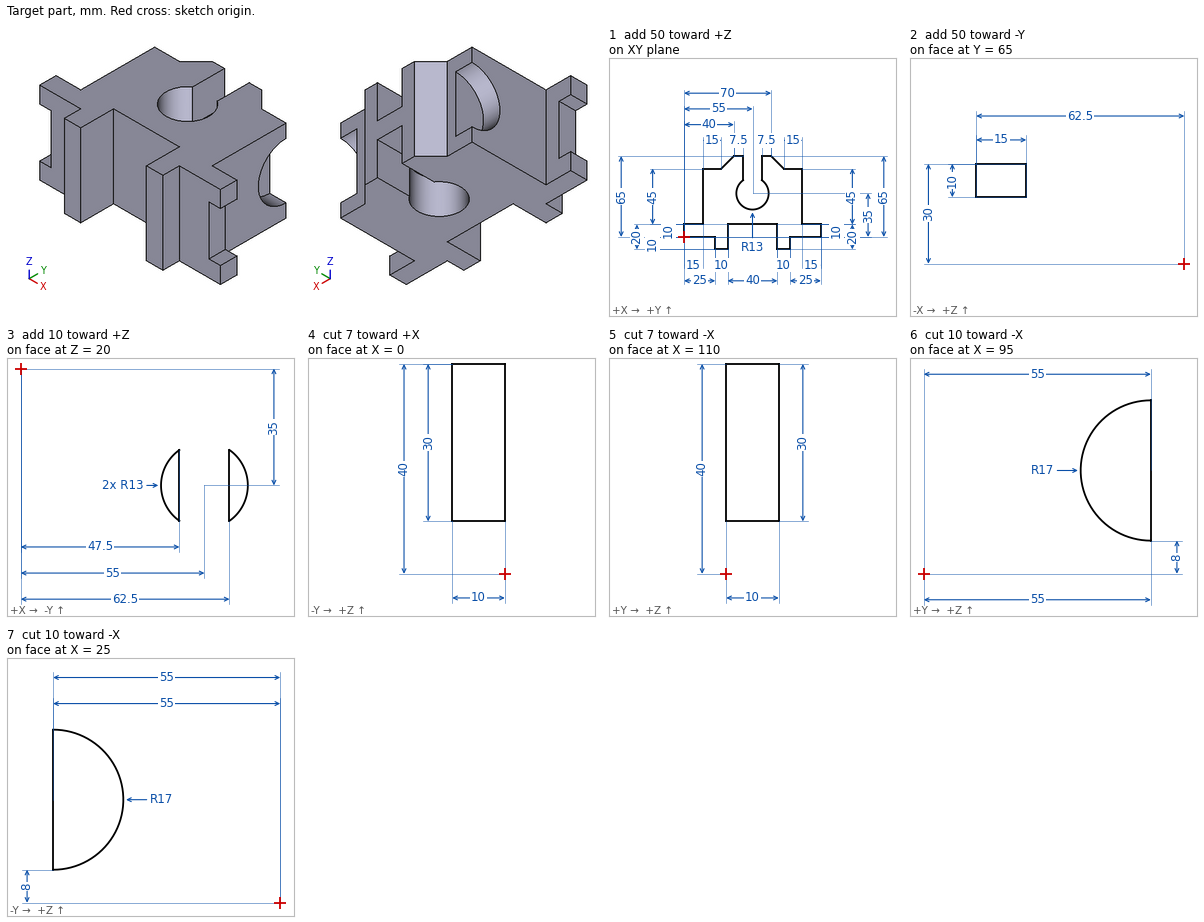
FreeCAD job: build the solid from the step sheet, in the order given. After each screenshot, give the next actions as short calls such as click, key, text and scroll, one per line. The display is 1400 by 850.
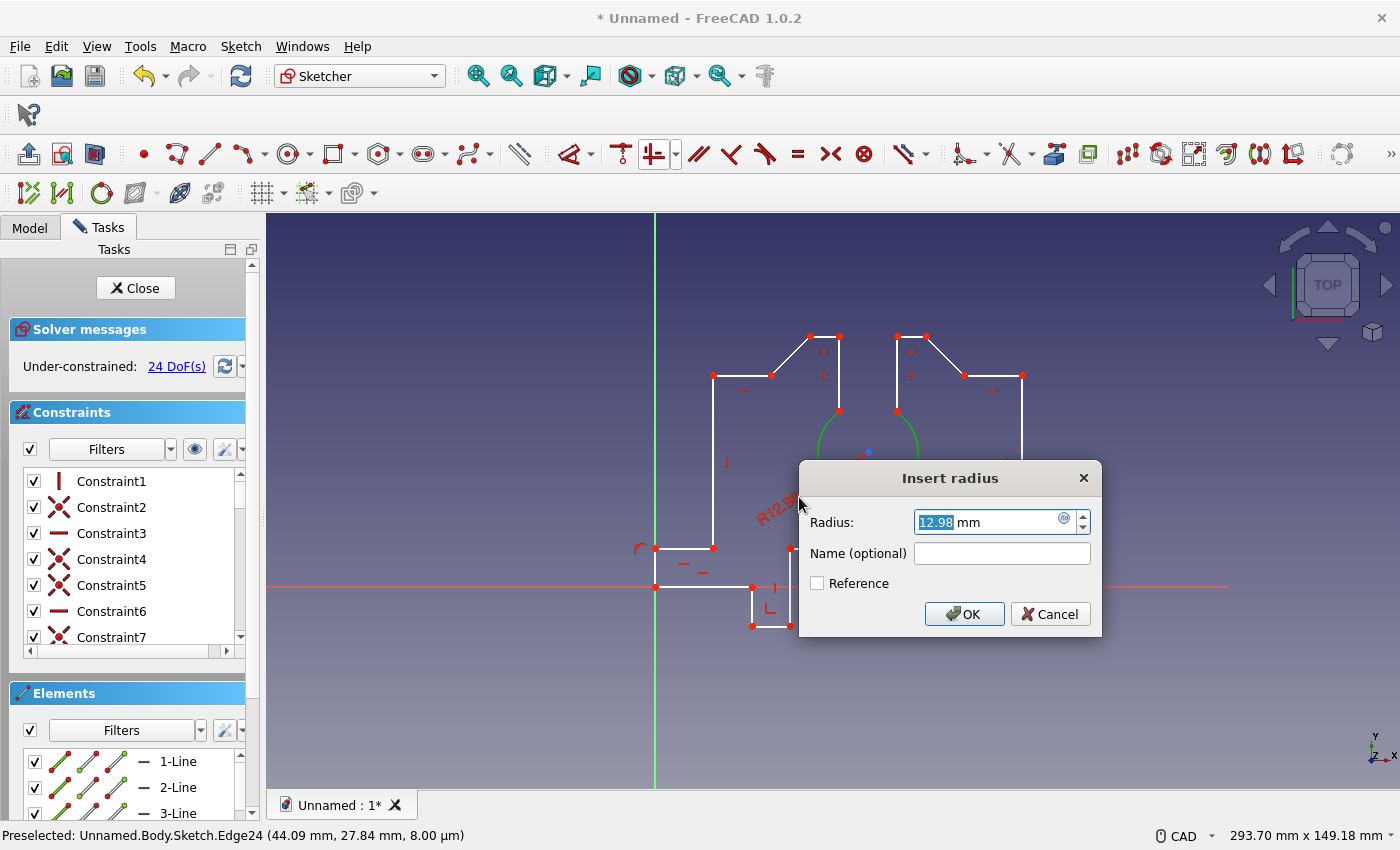
text(13)
key(Return)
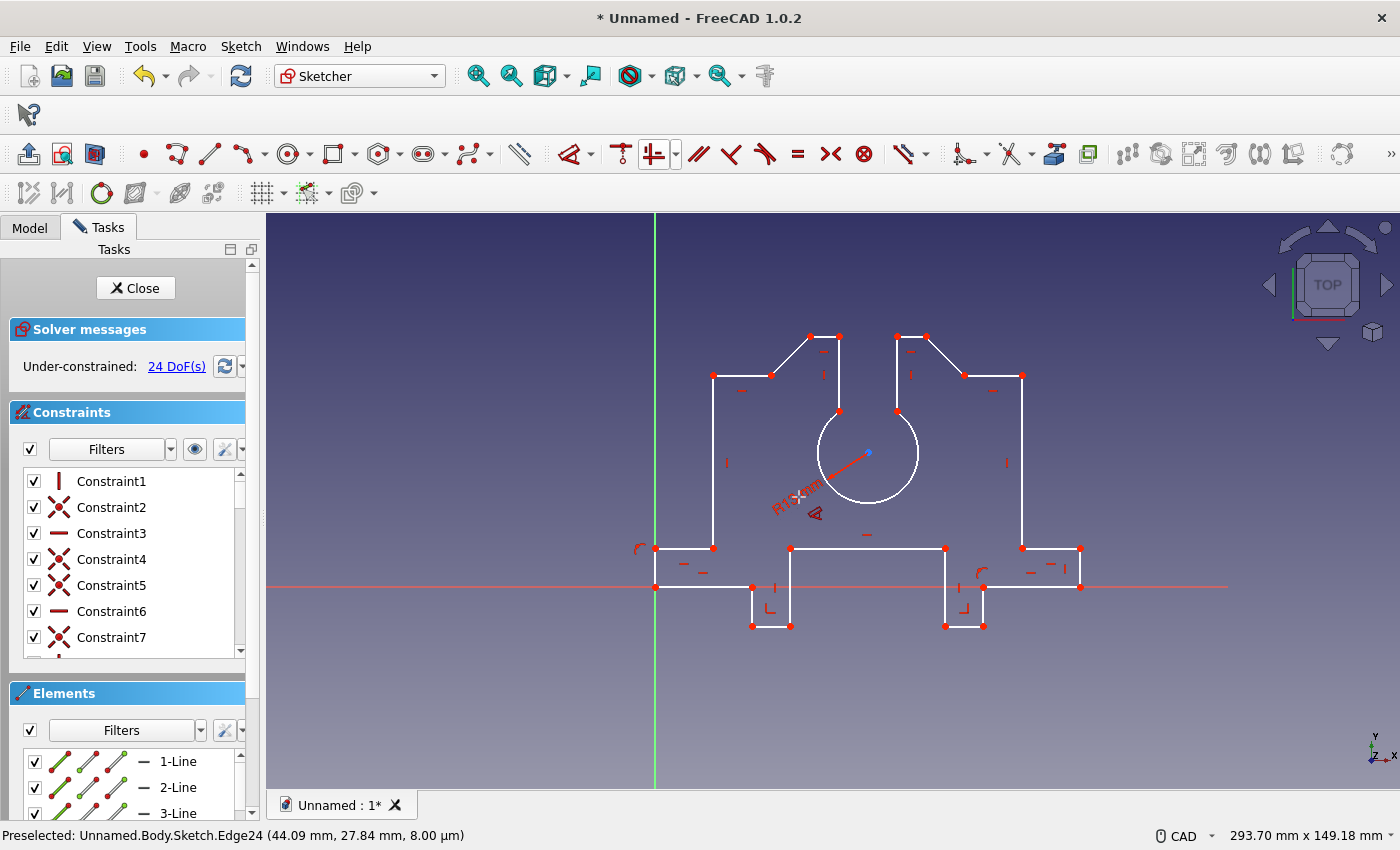
click(754, 376)
click(742, 342)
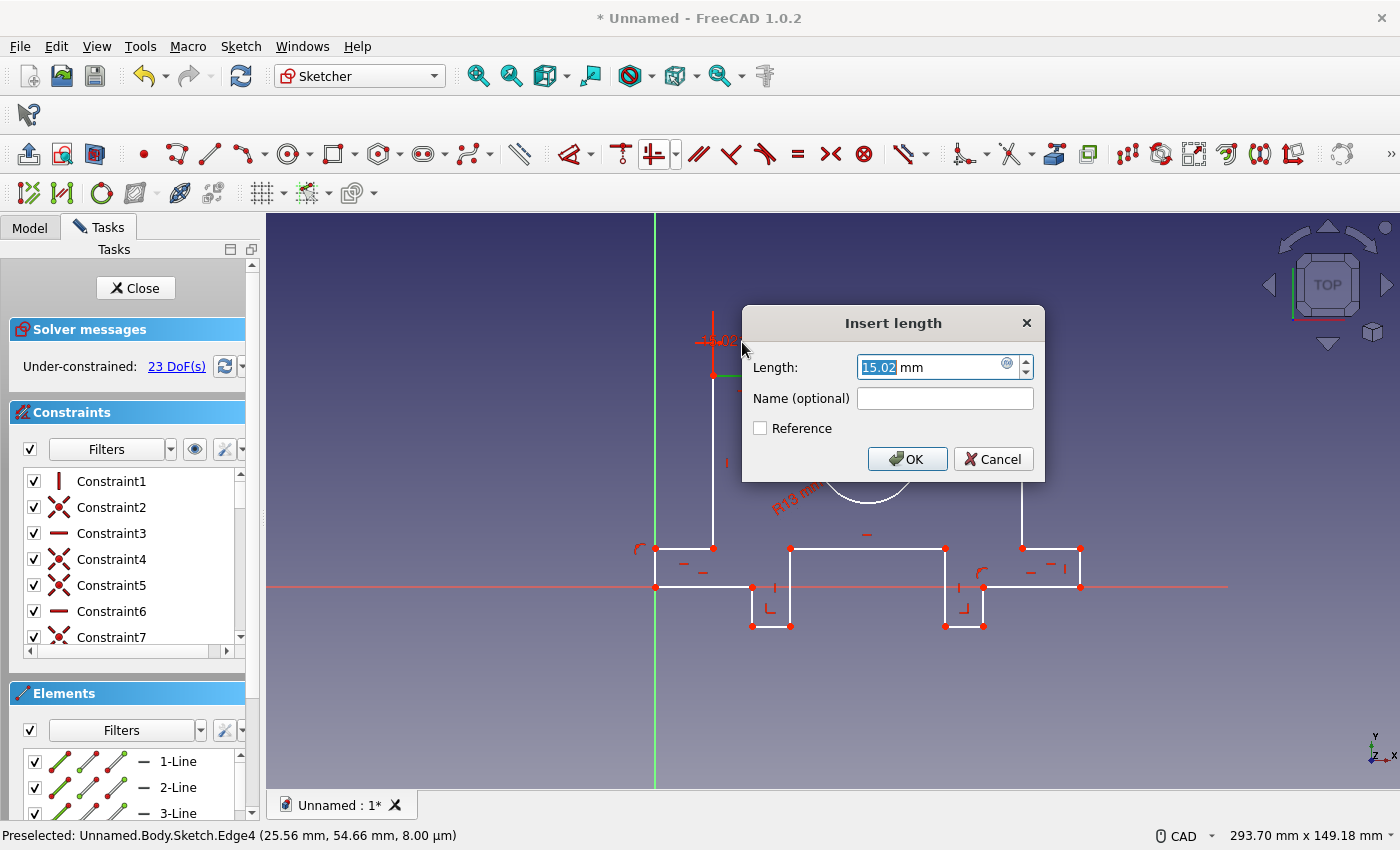
text(15)
key(Return)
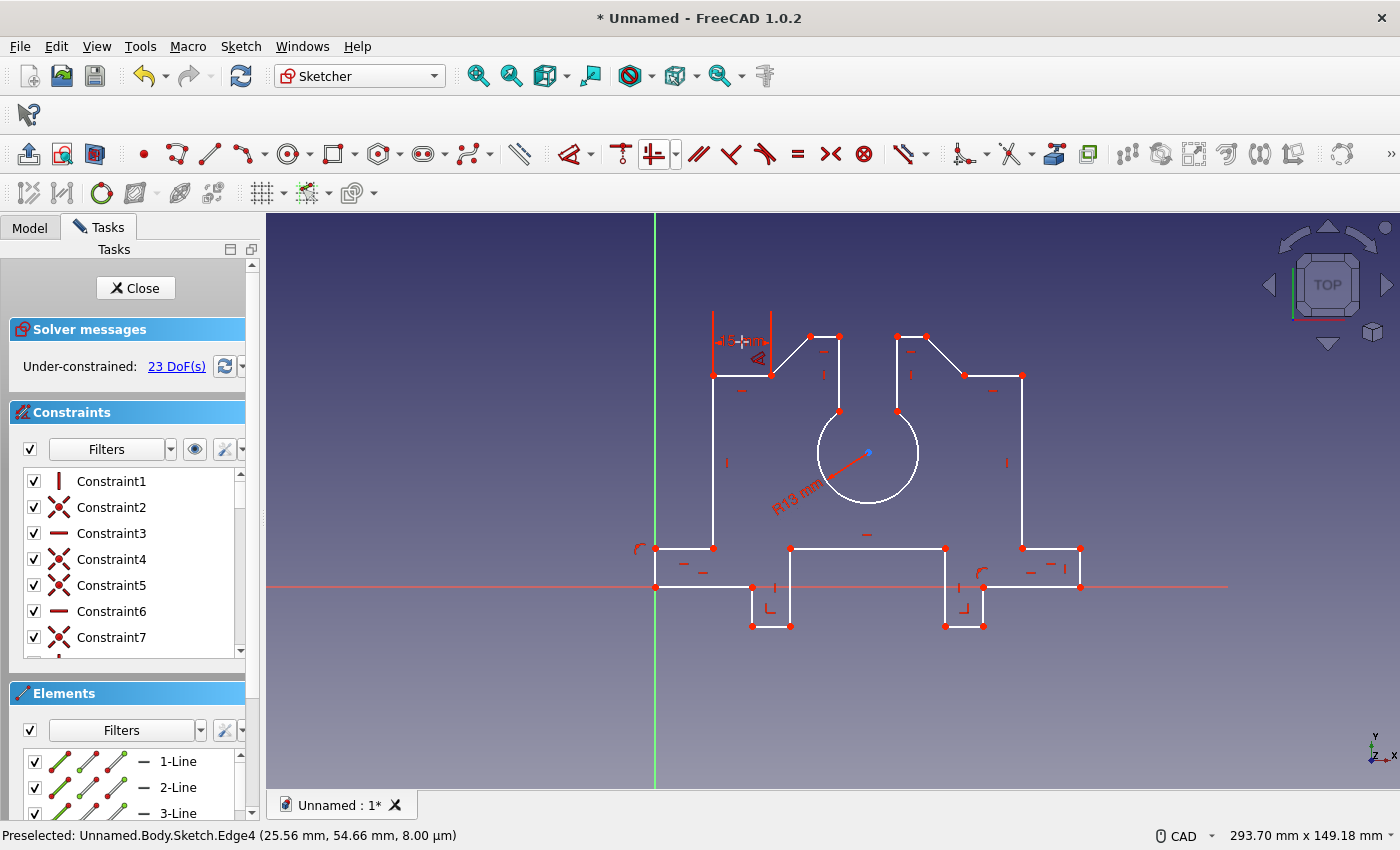
click(713, 428)
click(679, 463)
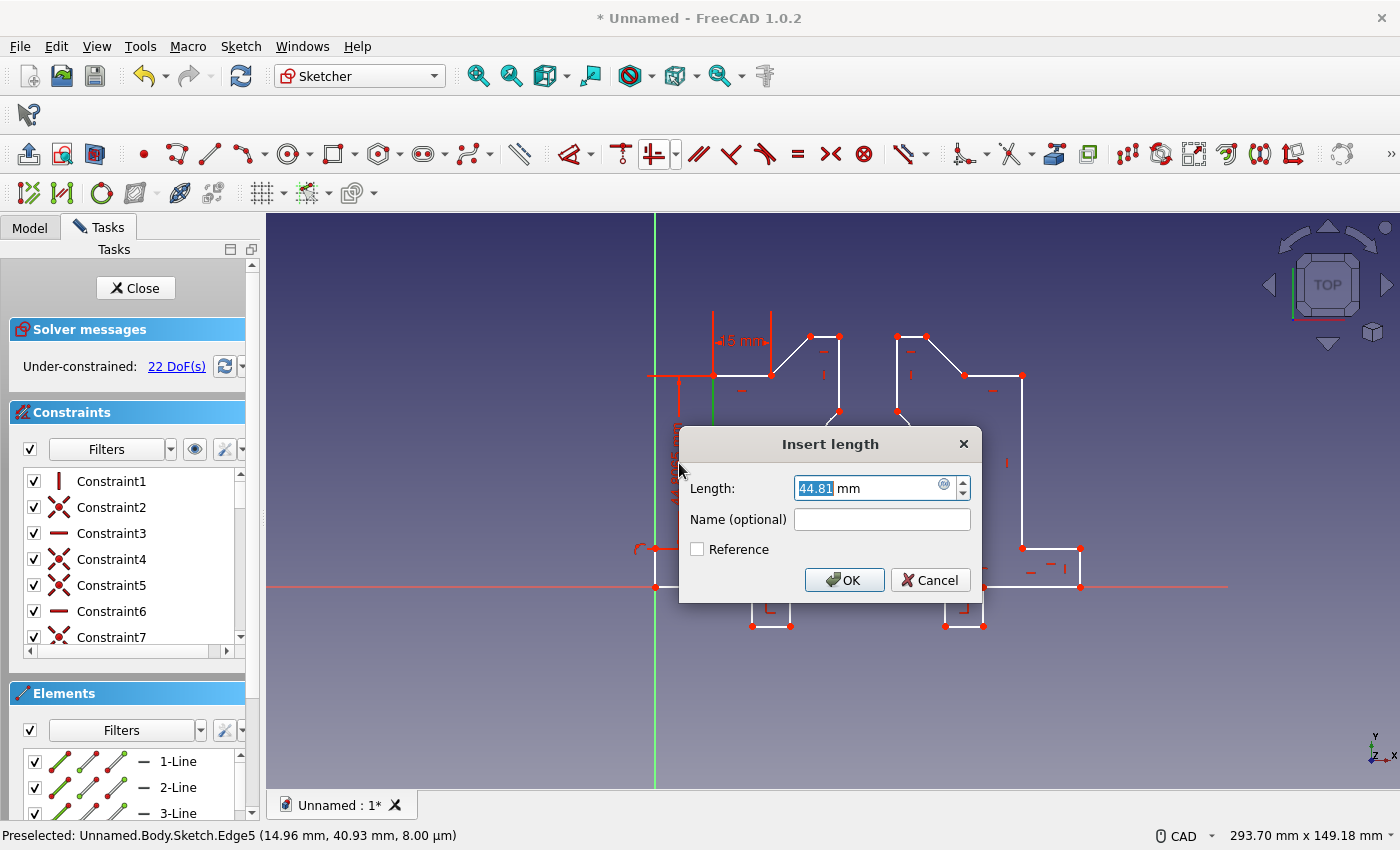
text(45)
key(Return)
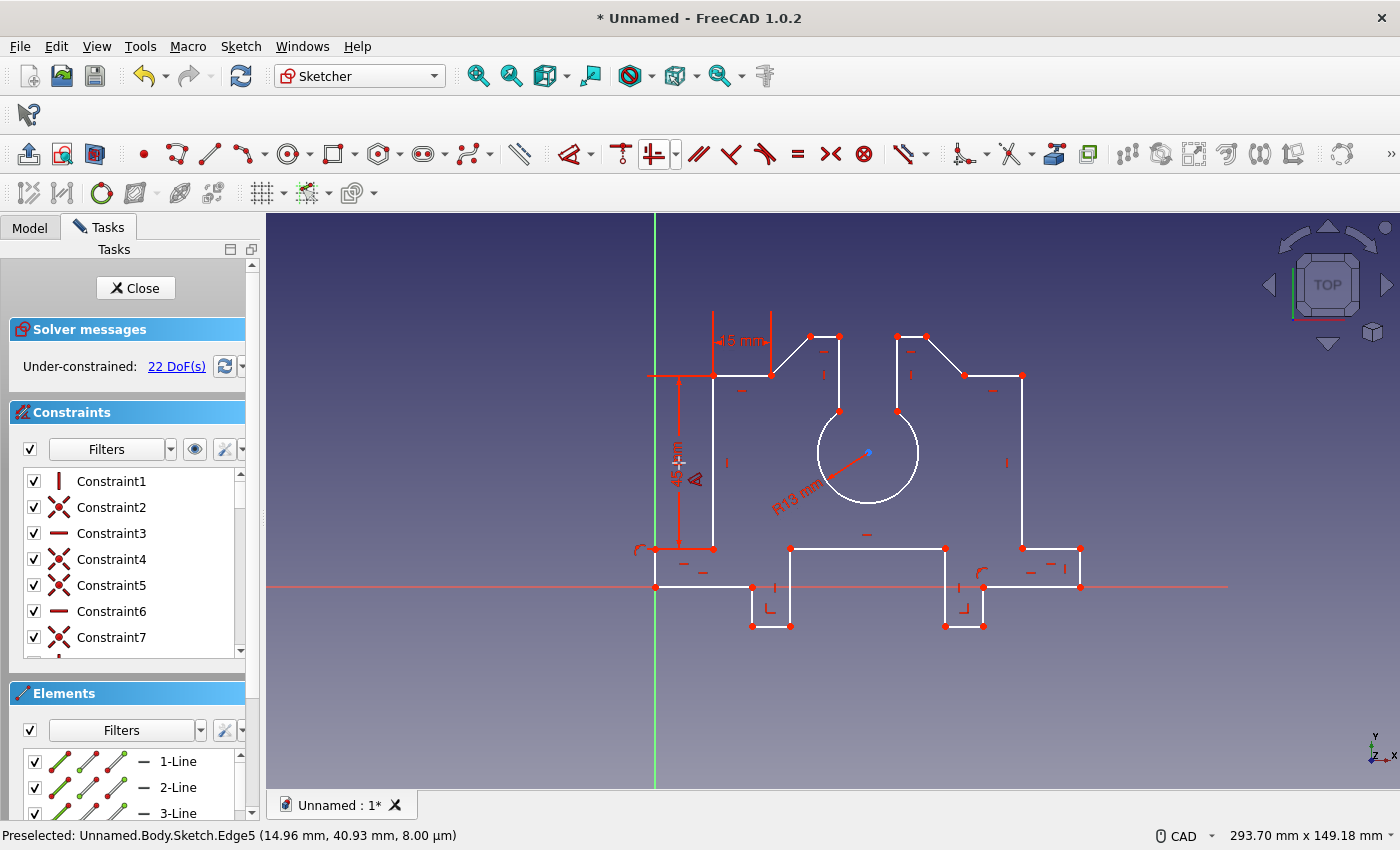
click(696, 549)
click(684, 515)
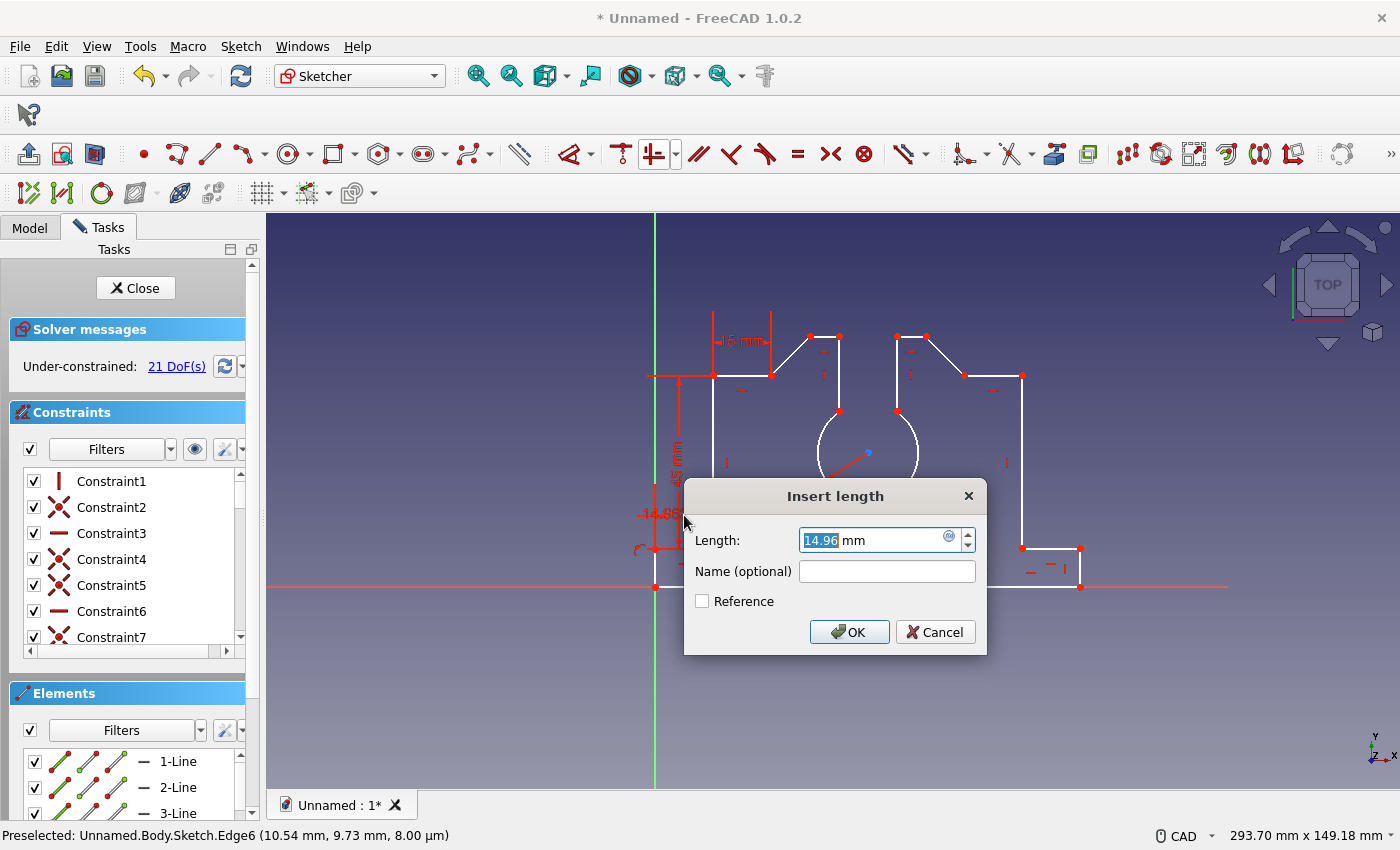
text(15)
key(Return)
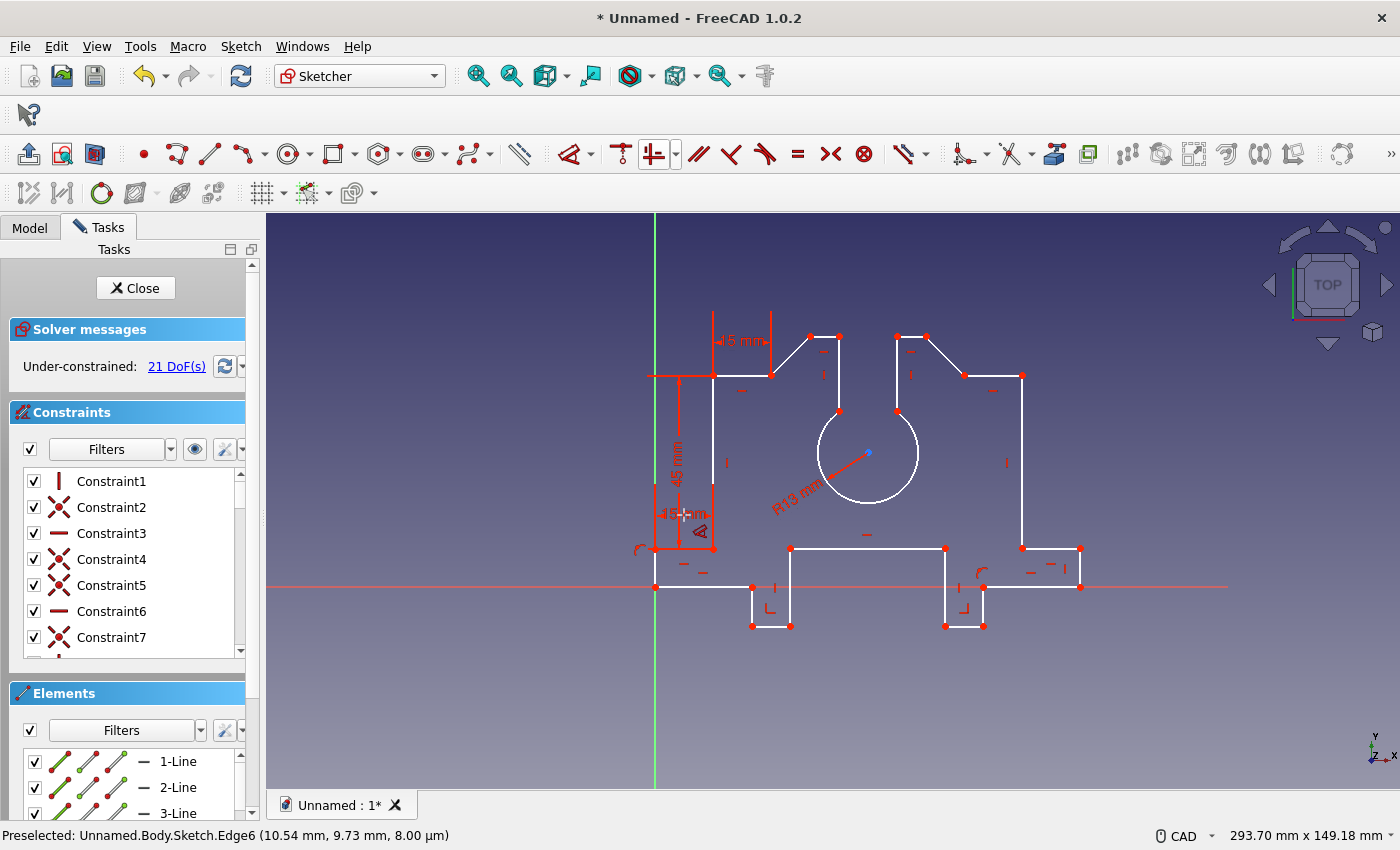
scroll(655, 561, up, 2)